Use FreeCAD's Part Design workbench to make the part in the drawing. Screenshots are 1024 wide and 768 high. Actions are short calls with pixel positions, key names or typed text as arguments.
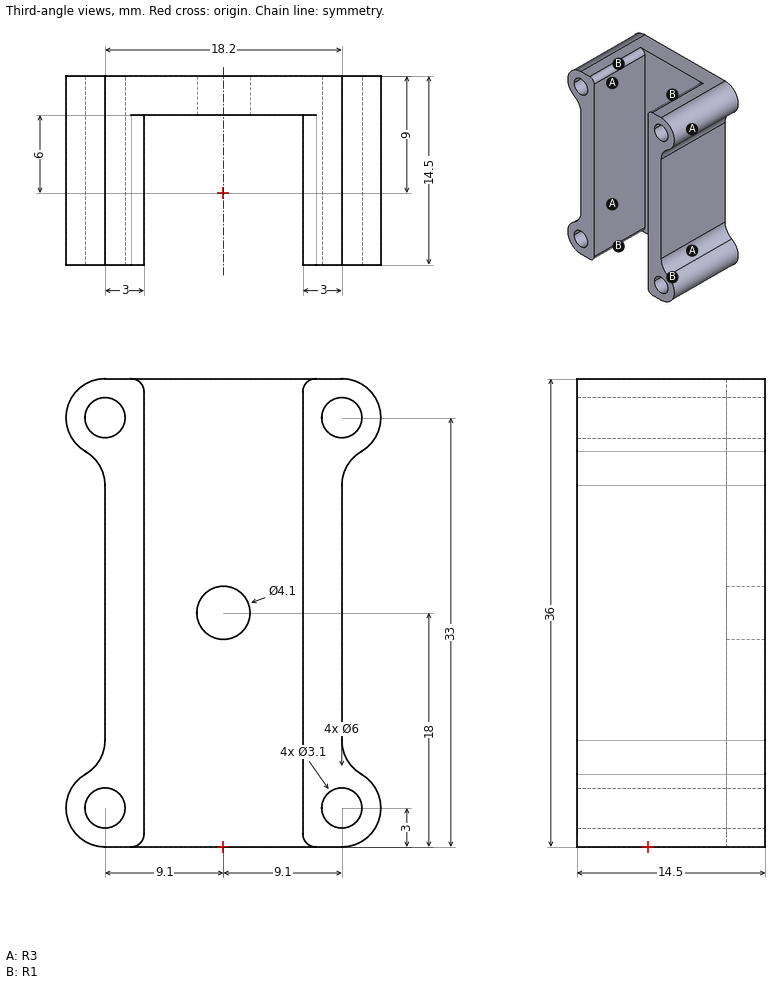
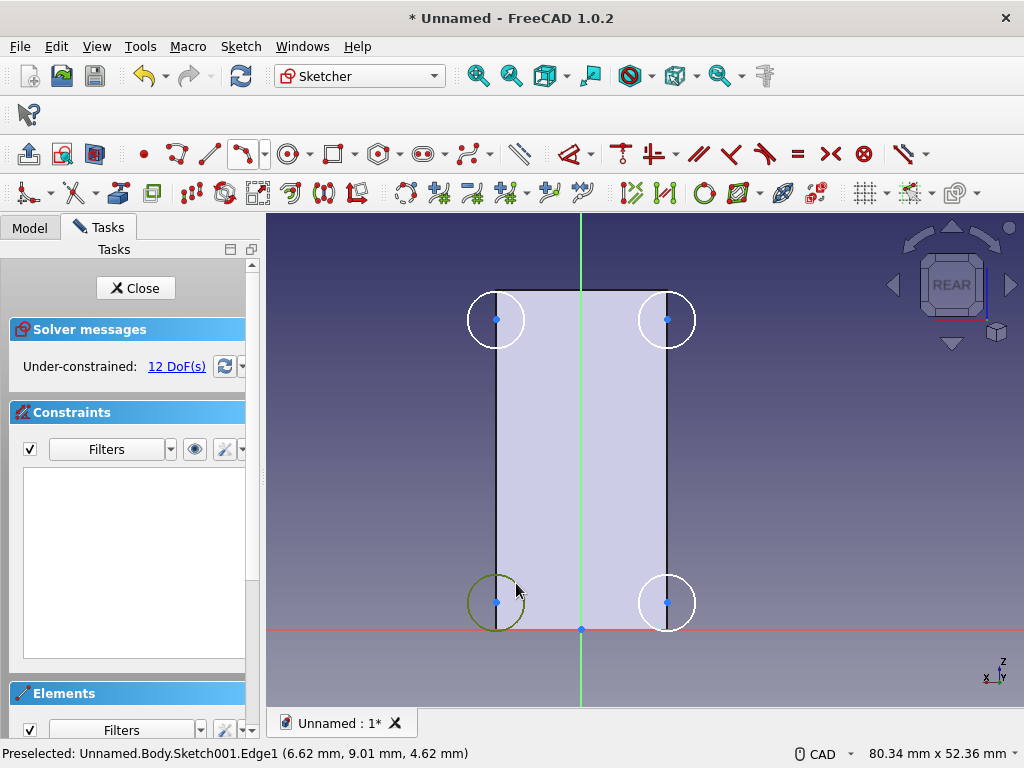
click(687, 583)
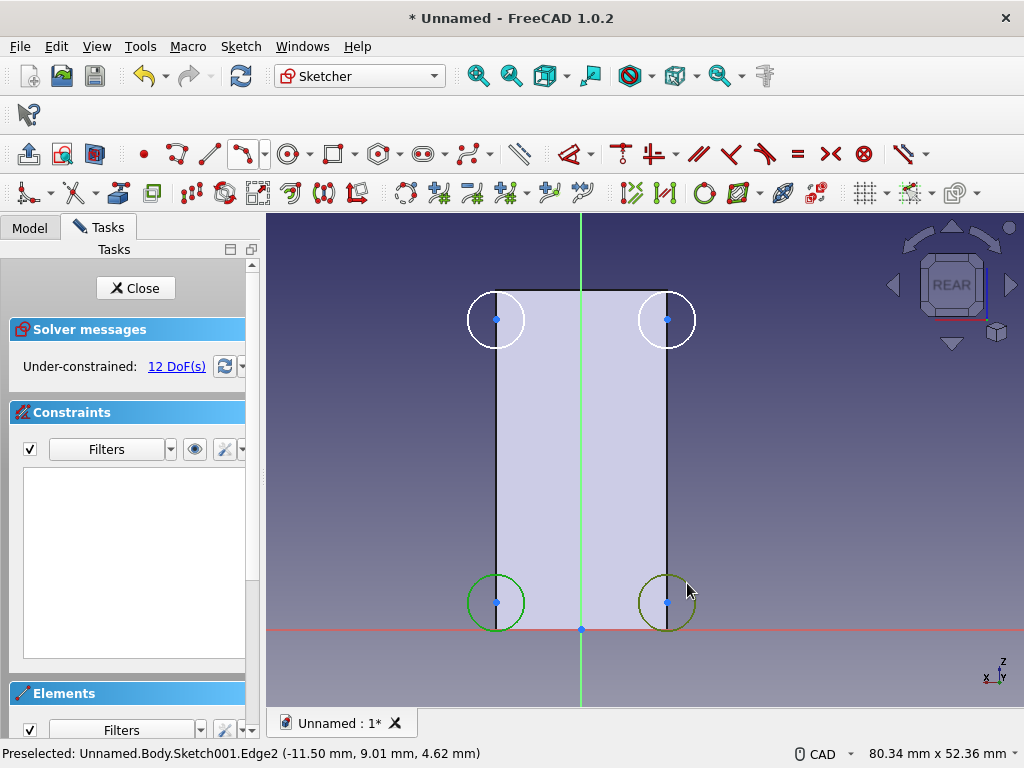
click(516, 300)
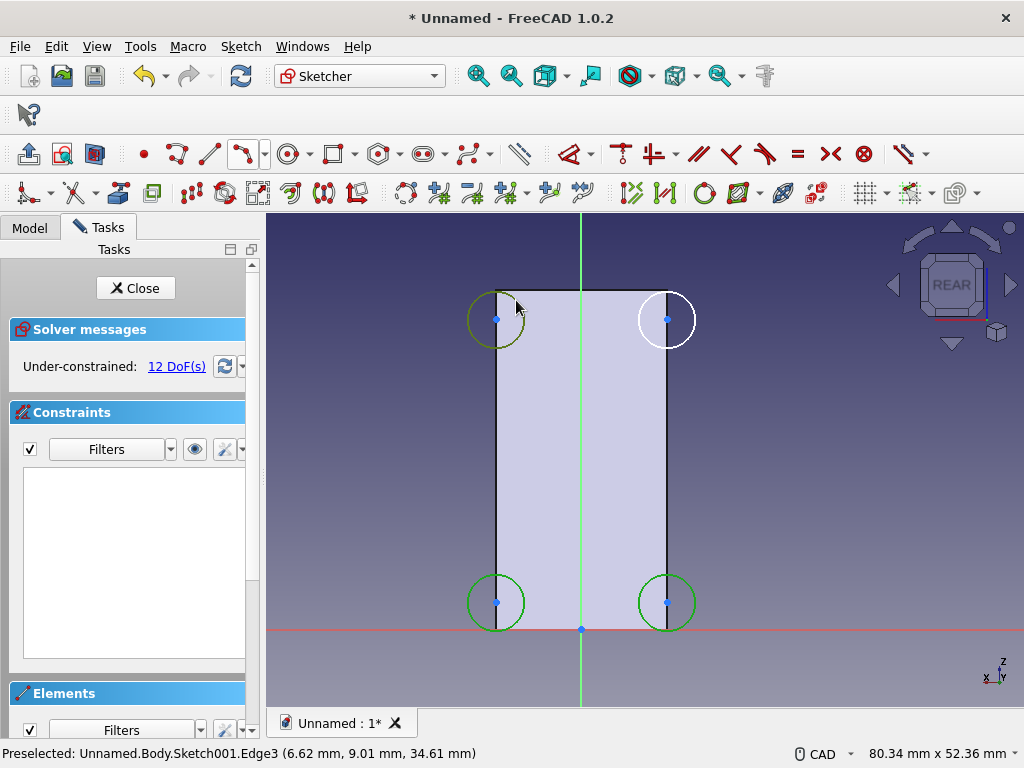
click(687, 300)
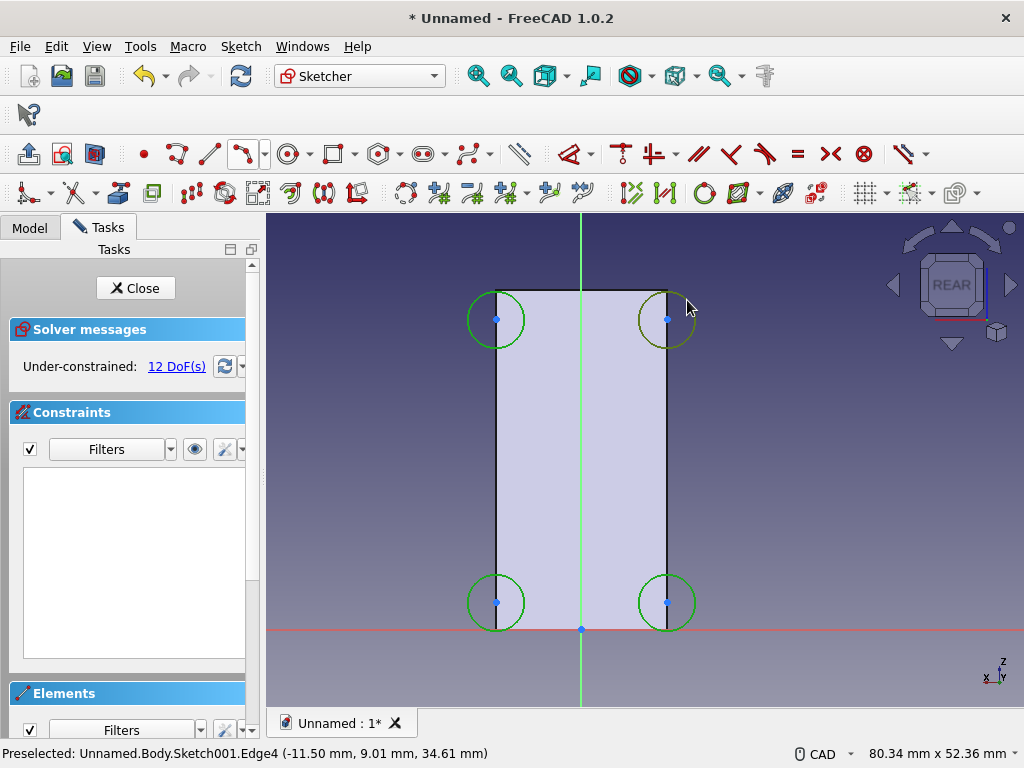
click(798, 154)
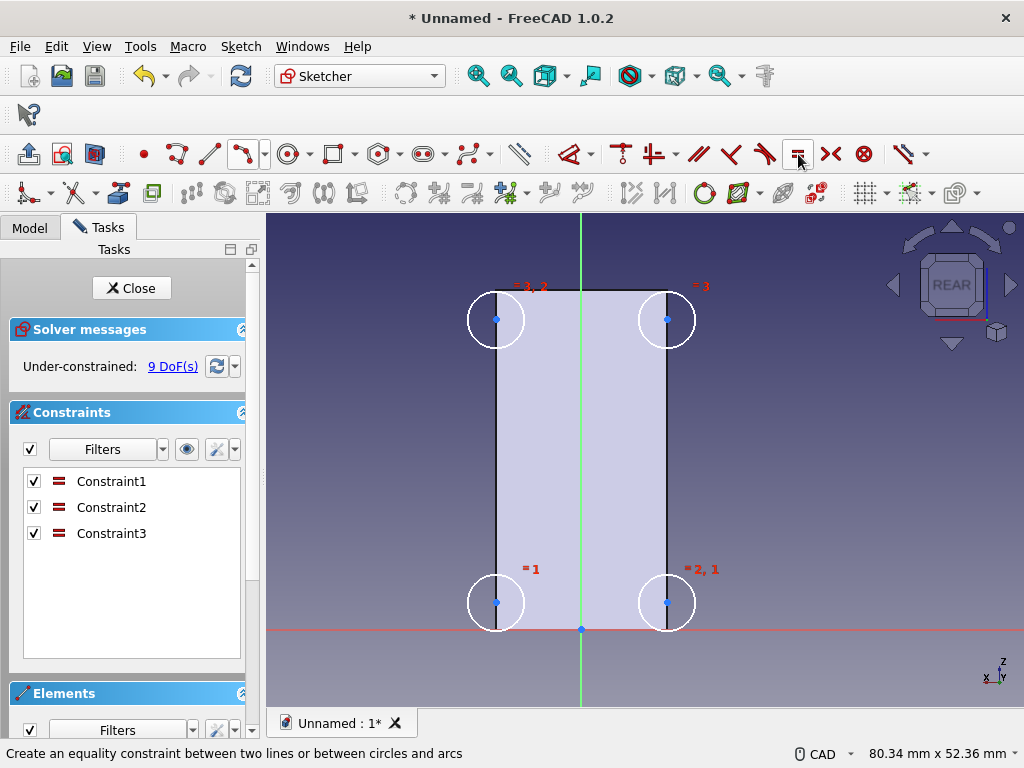
click(496, 603)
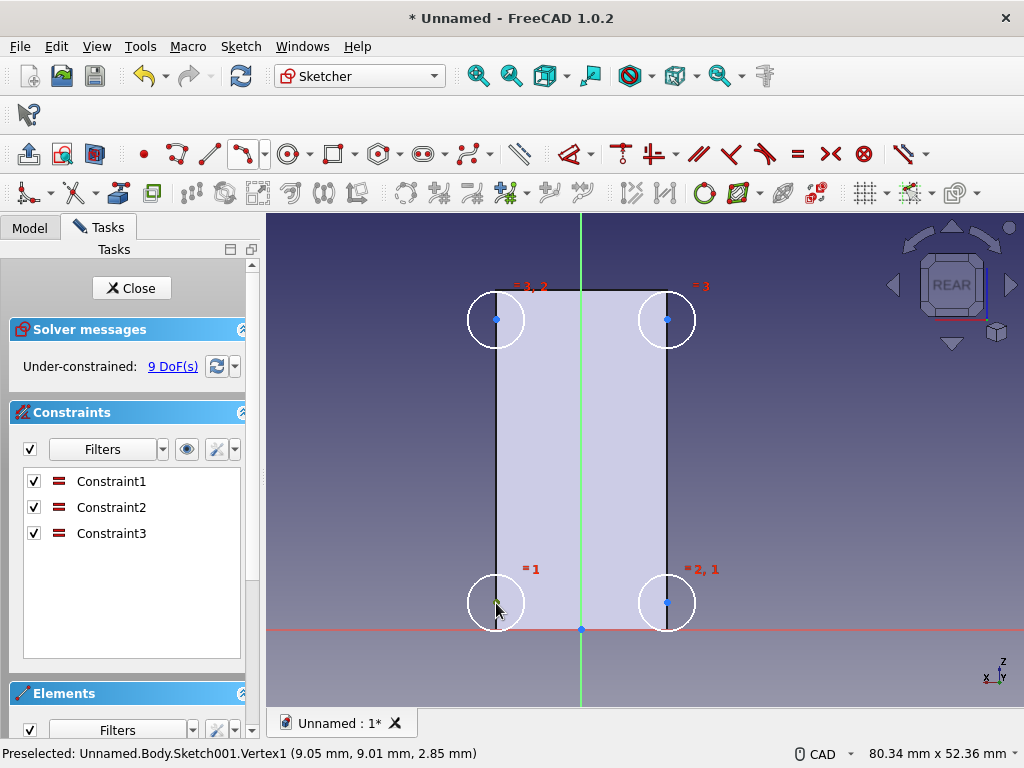
click(667, 603)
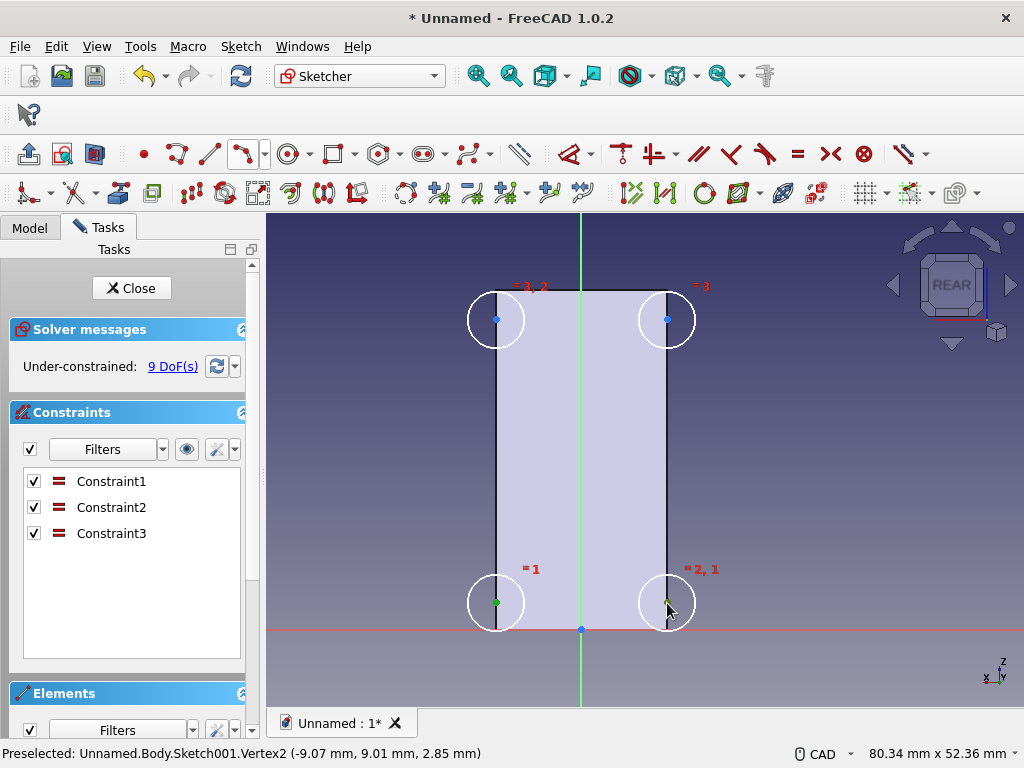
click(676, 154)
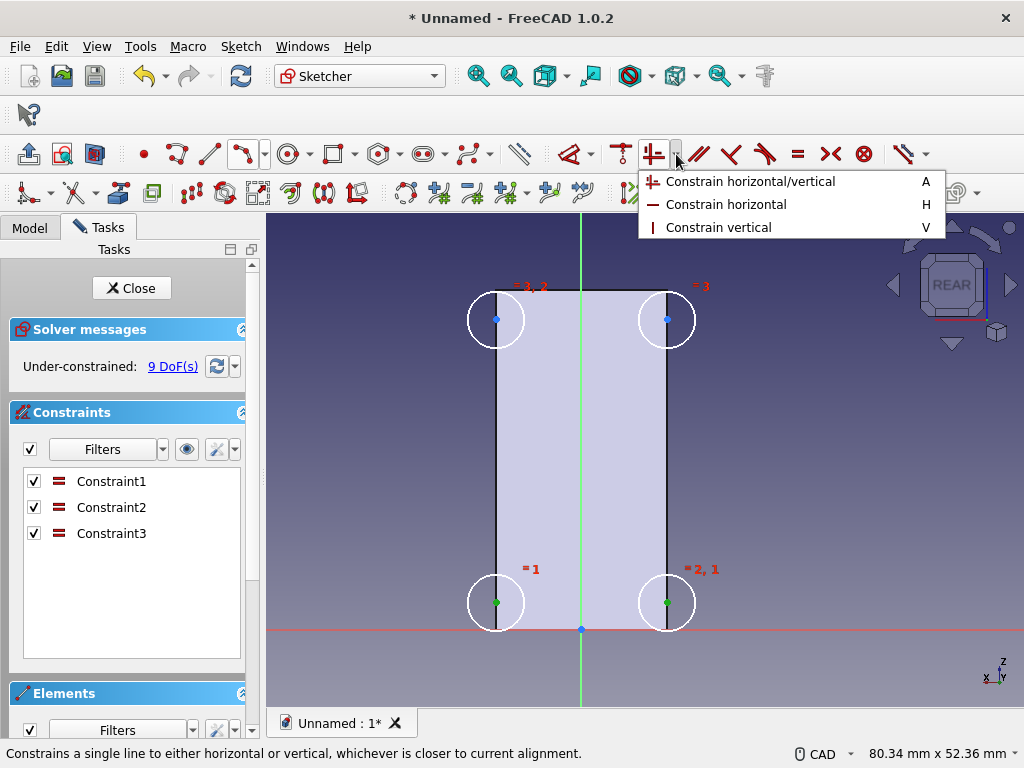
click(792, 204)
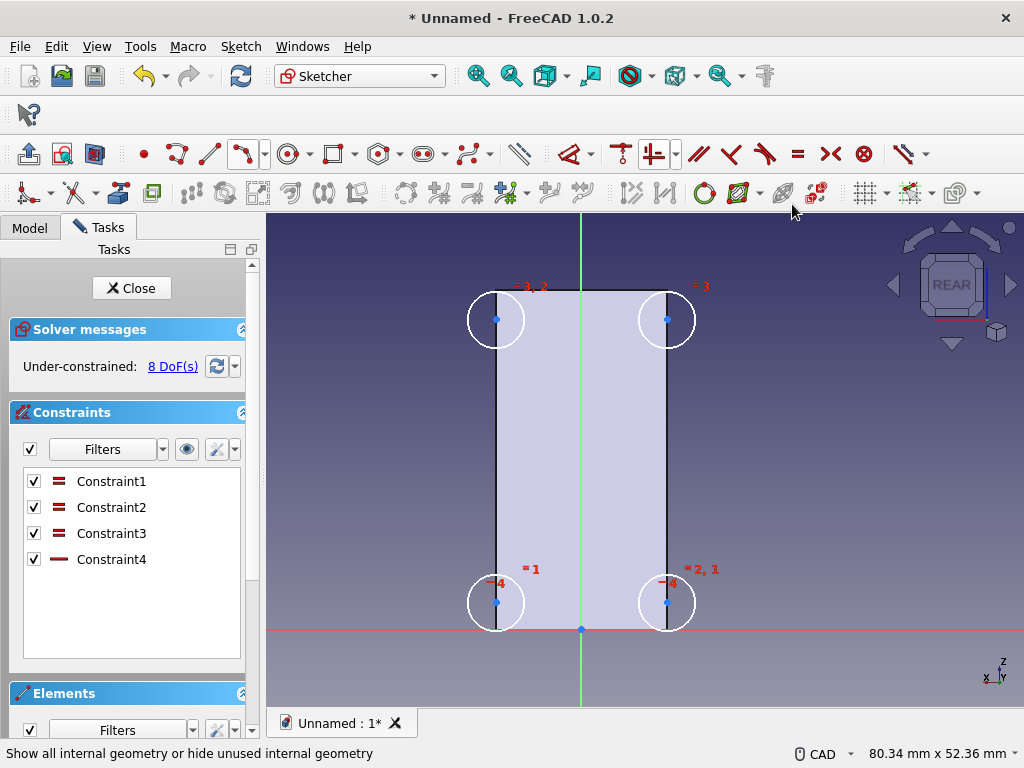
click(496, 603)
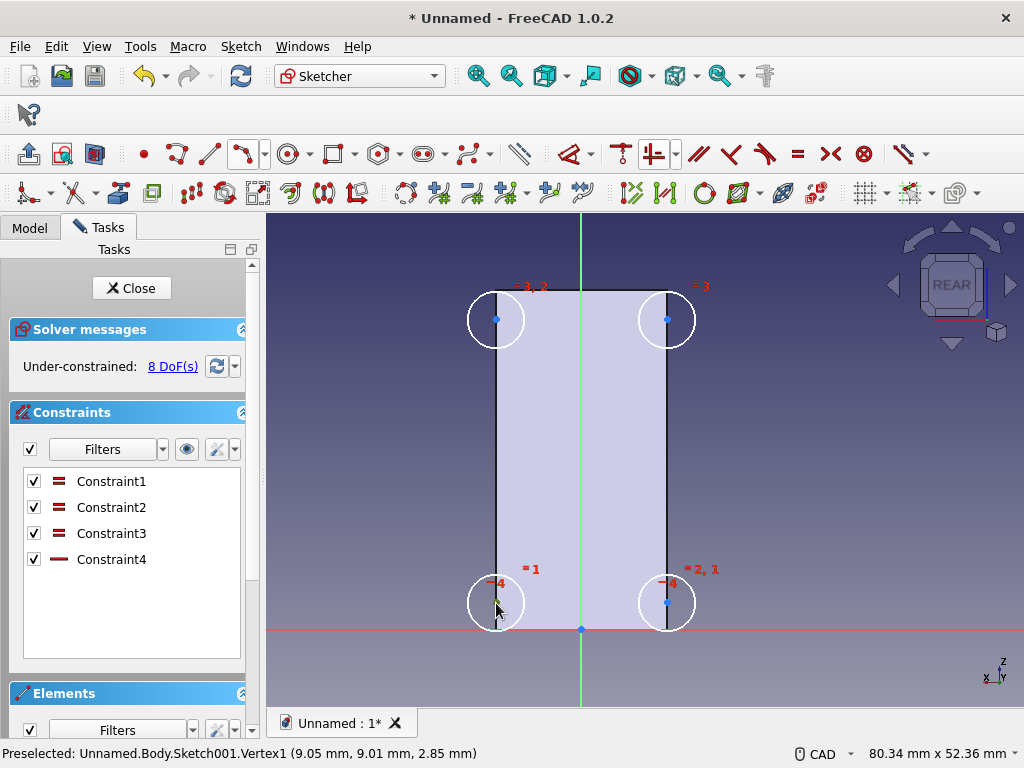
click(496, 320)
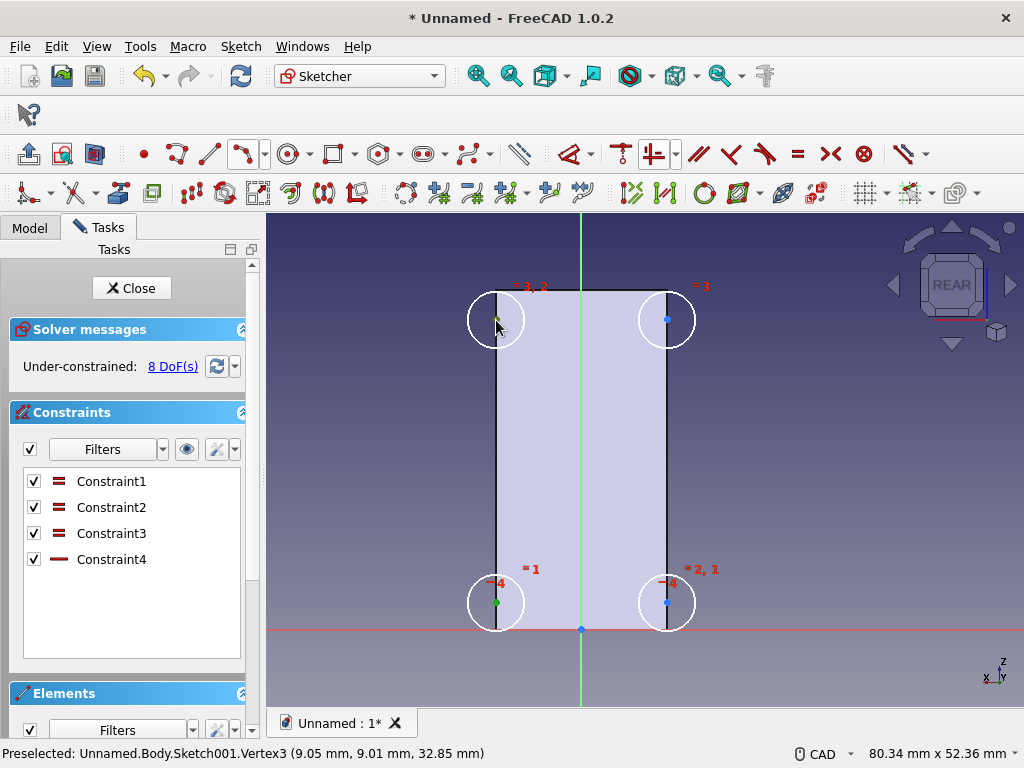
click(676, 154)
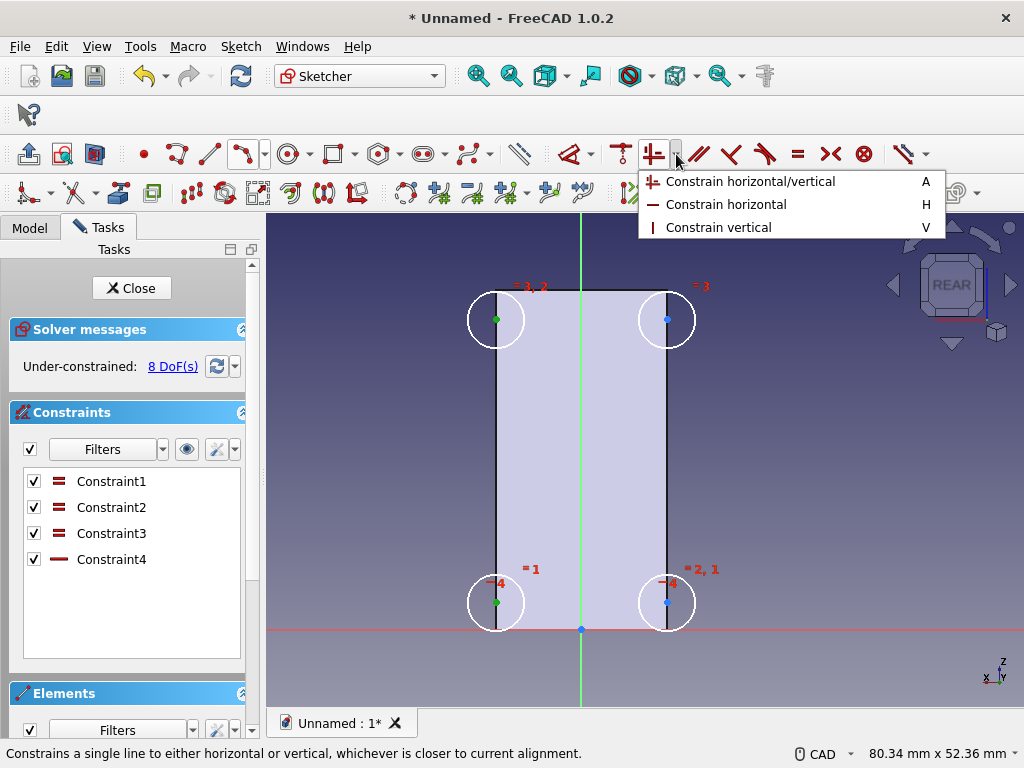
click(792, 228)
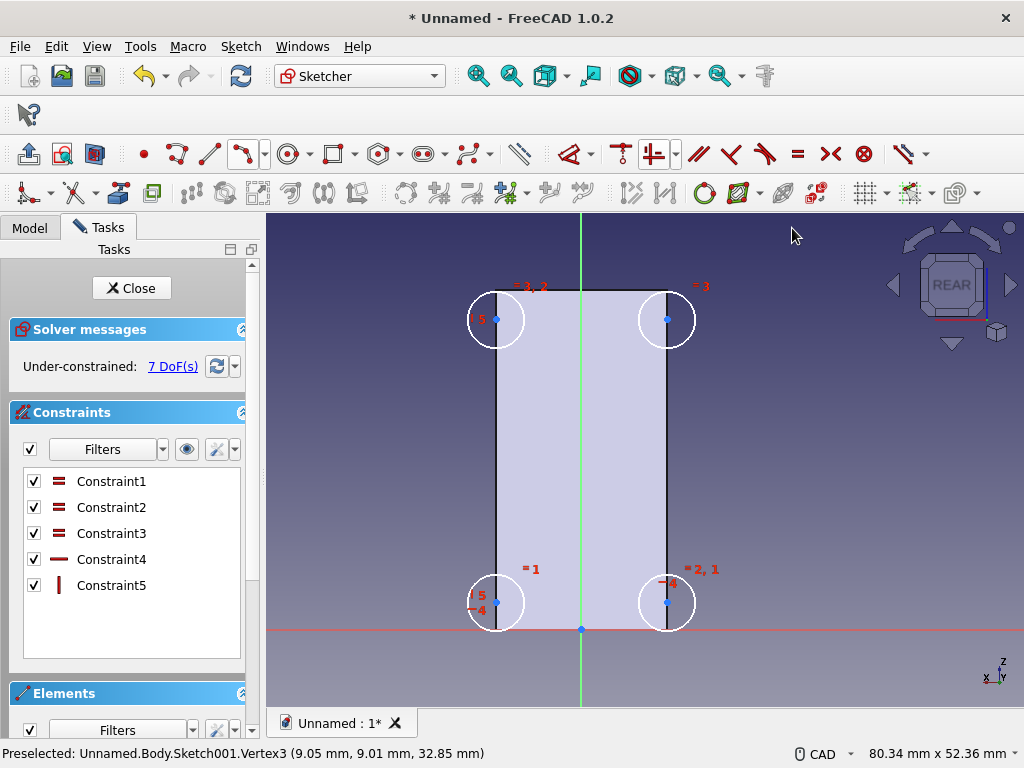
click(667, 603)